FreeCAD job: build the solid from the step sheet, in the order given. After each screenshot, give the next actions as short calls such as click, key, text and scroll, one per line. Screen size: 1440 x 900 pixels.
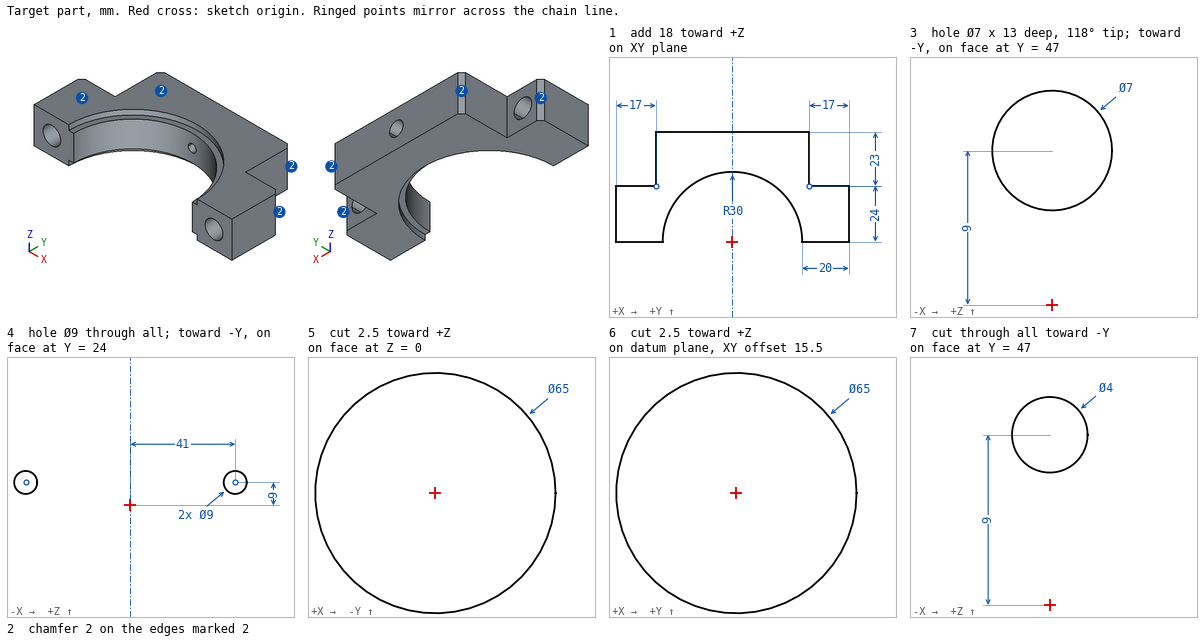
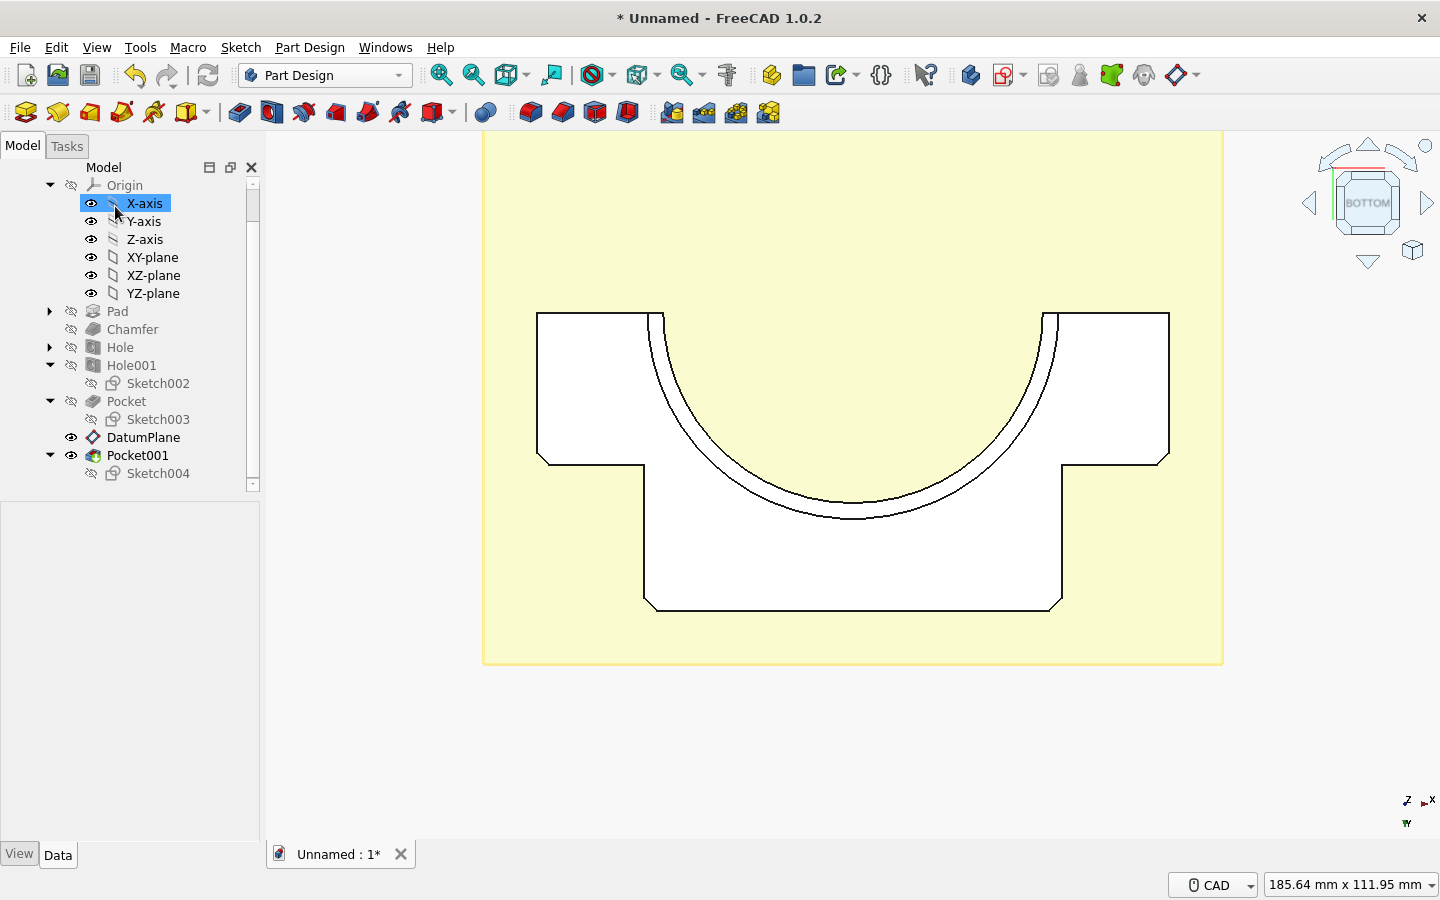
click(116, 437)
key(space)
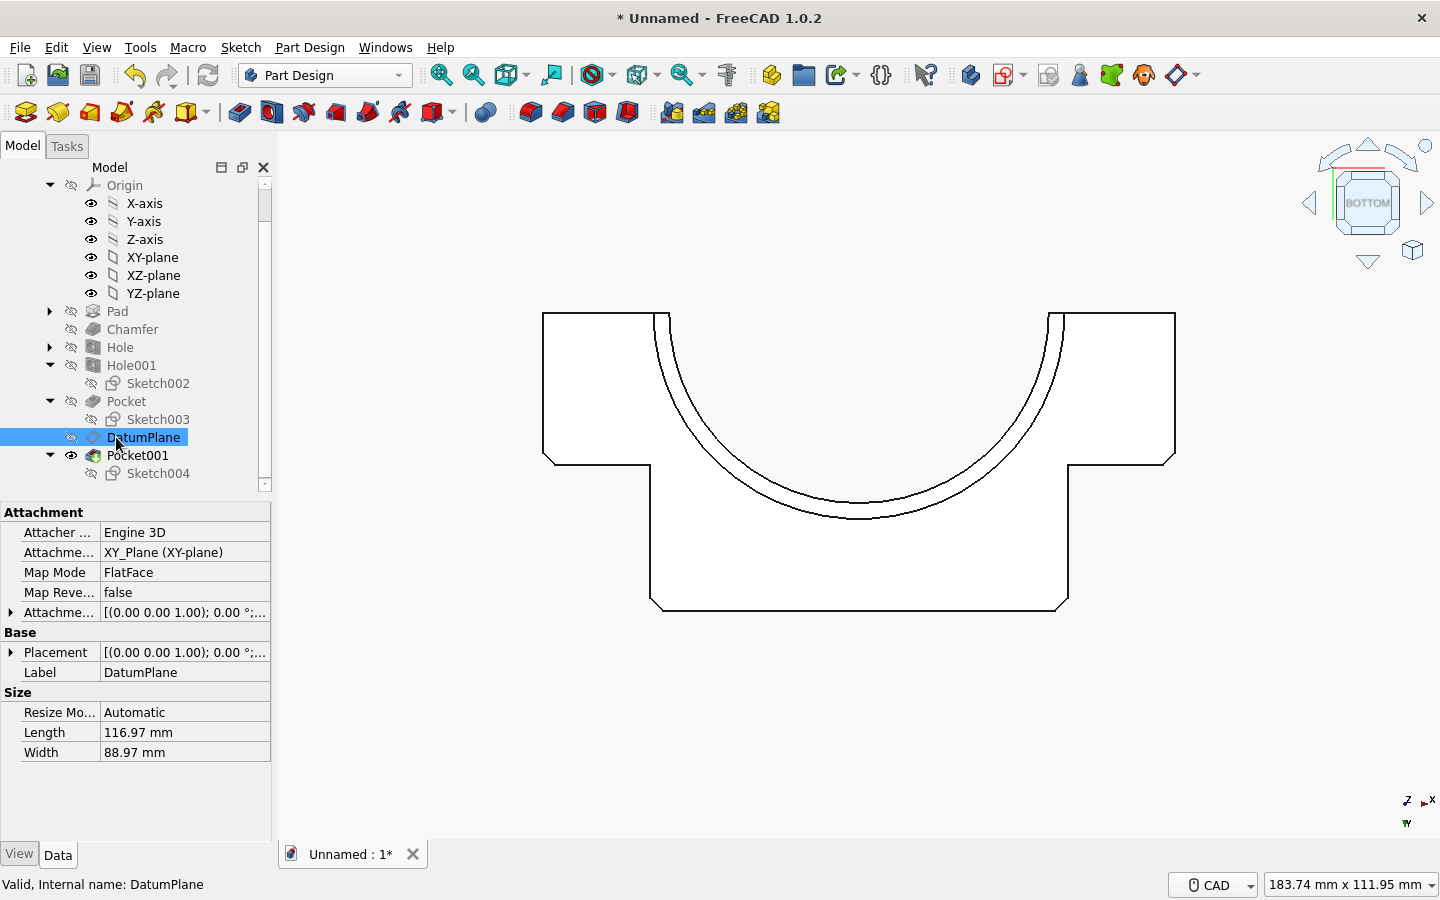
key(4)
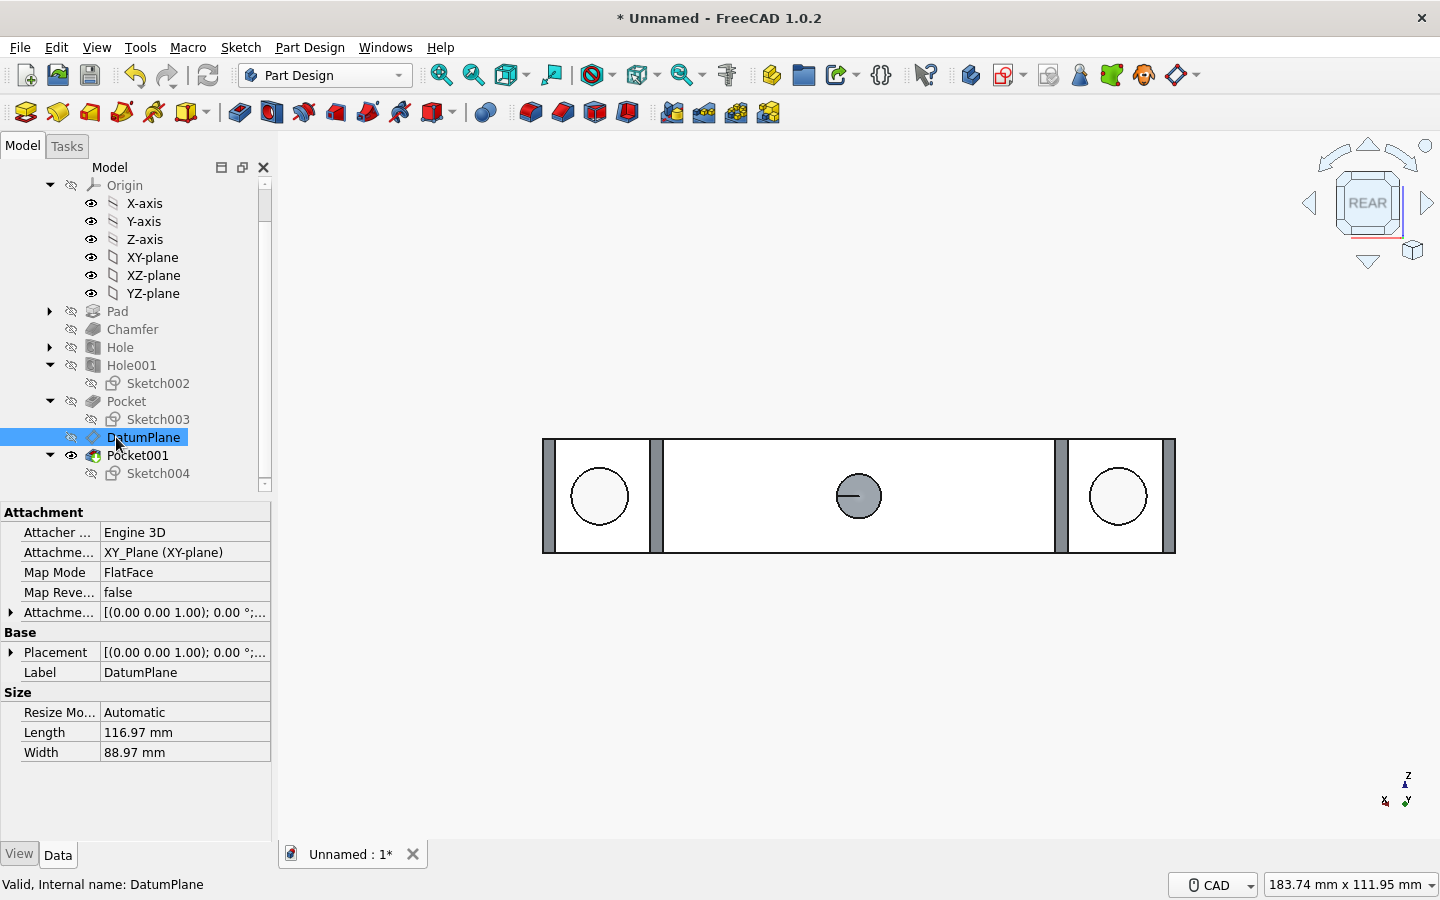
click(747, 495)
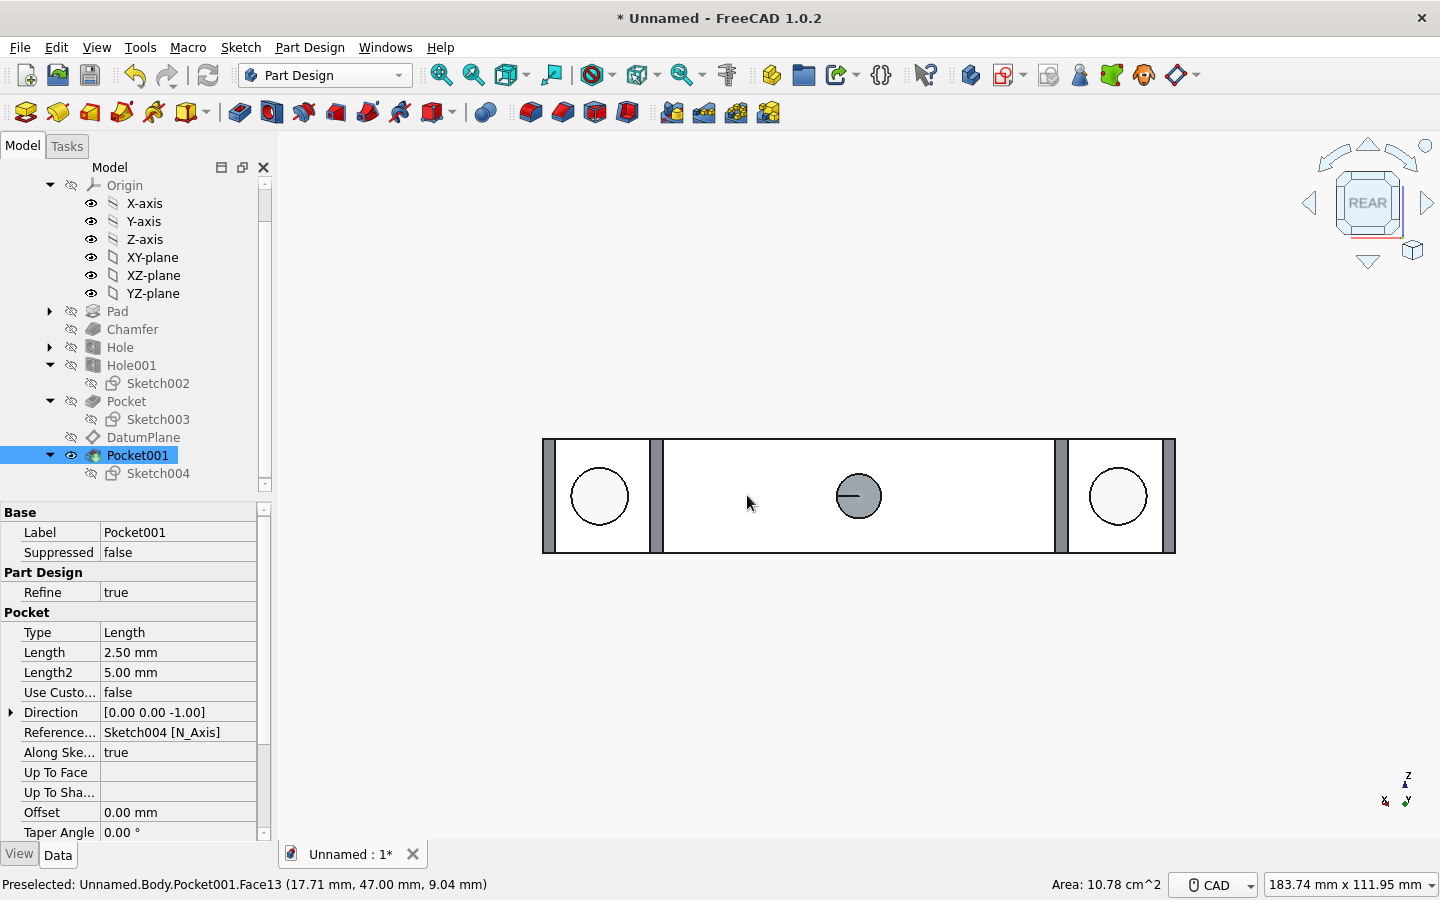
click(1004, 76)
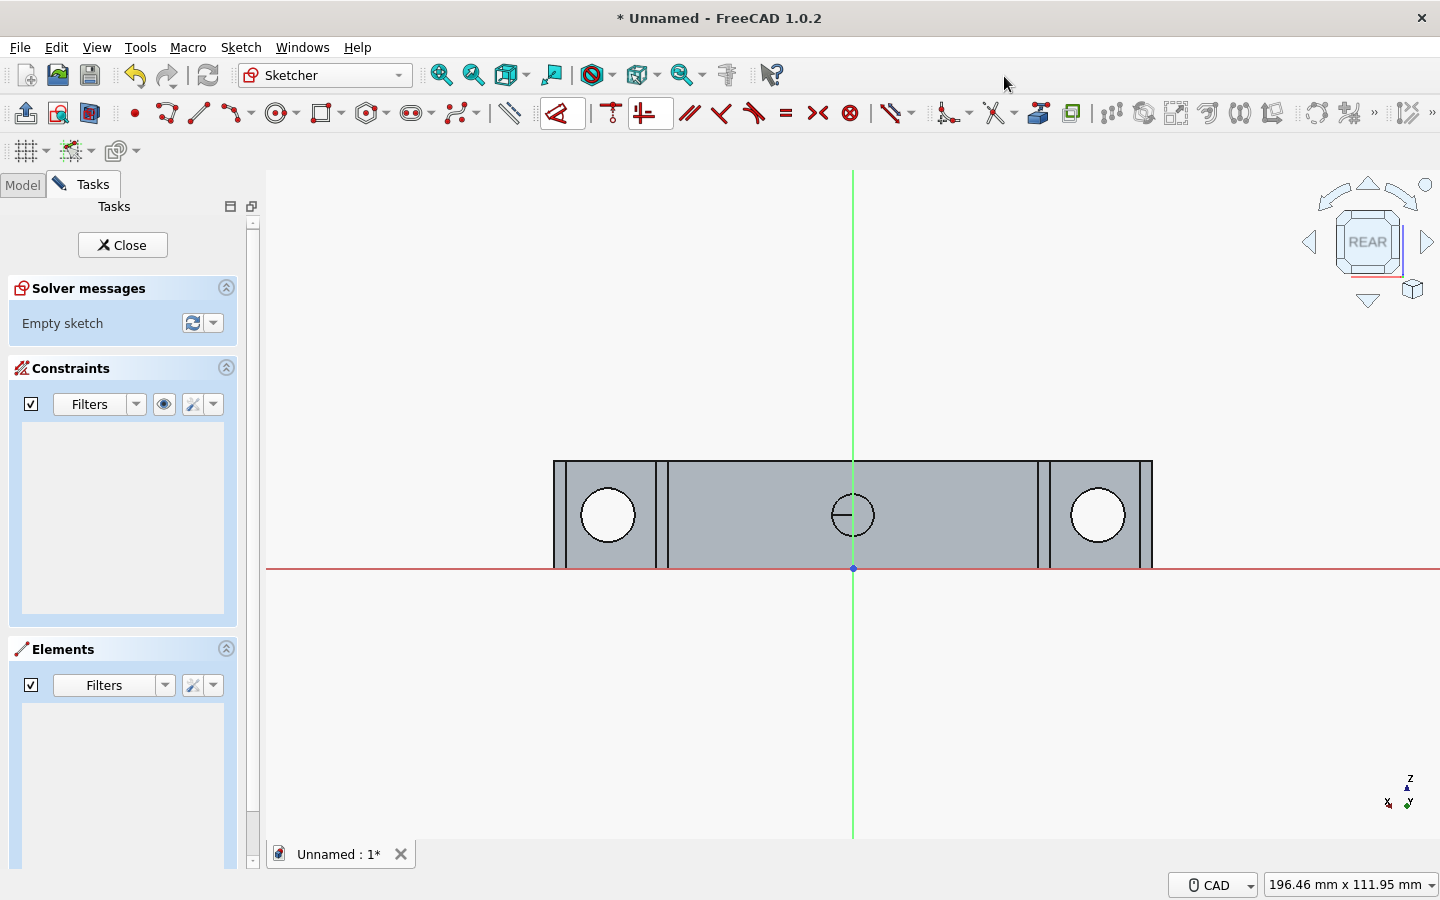
scroll(857, 516, up, 14)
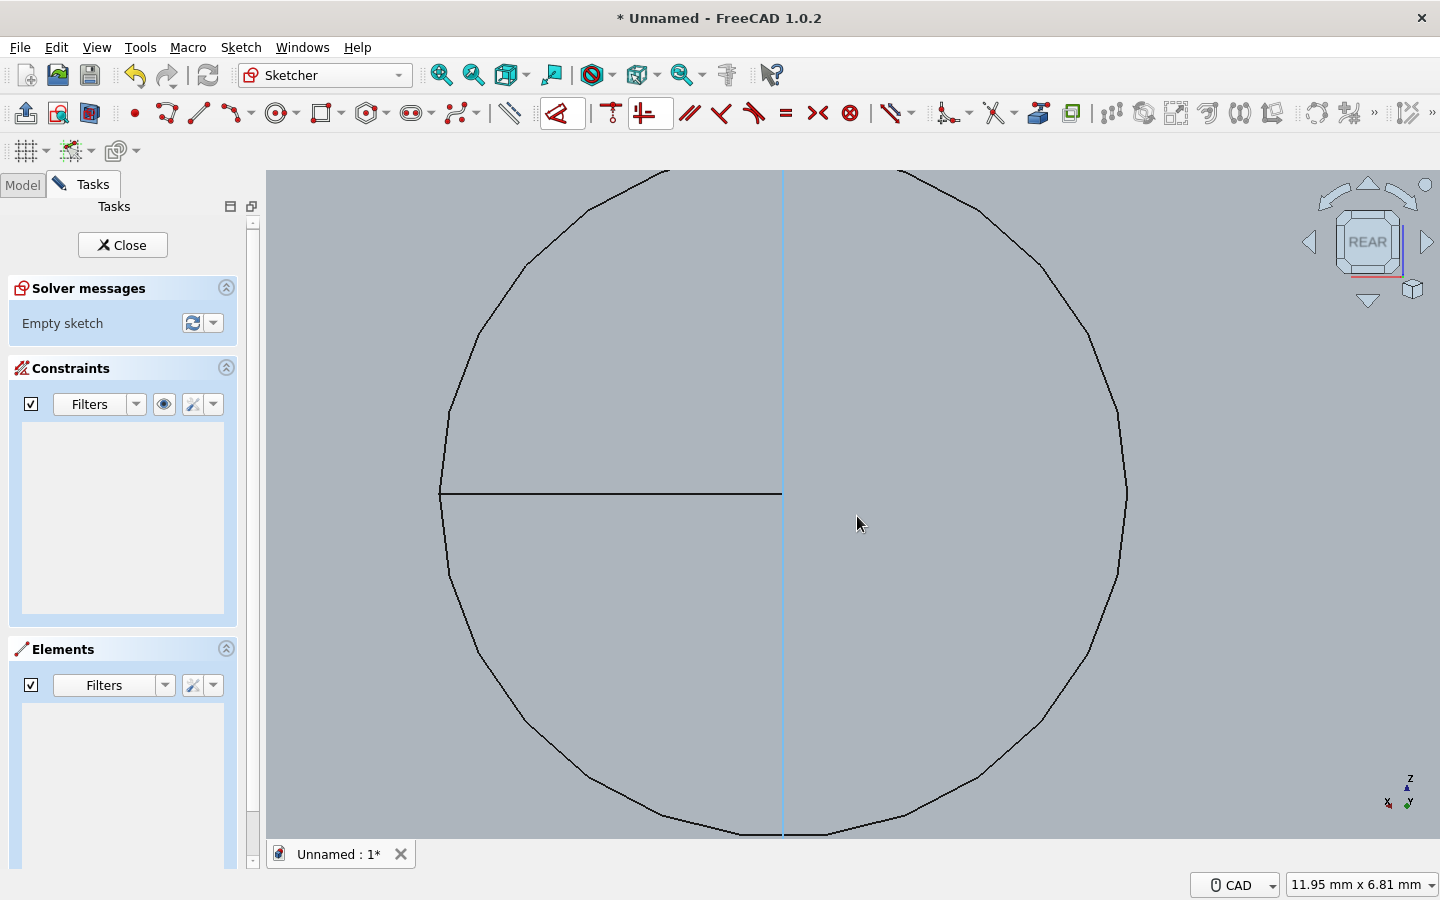
click(276, 114)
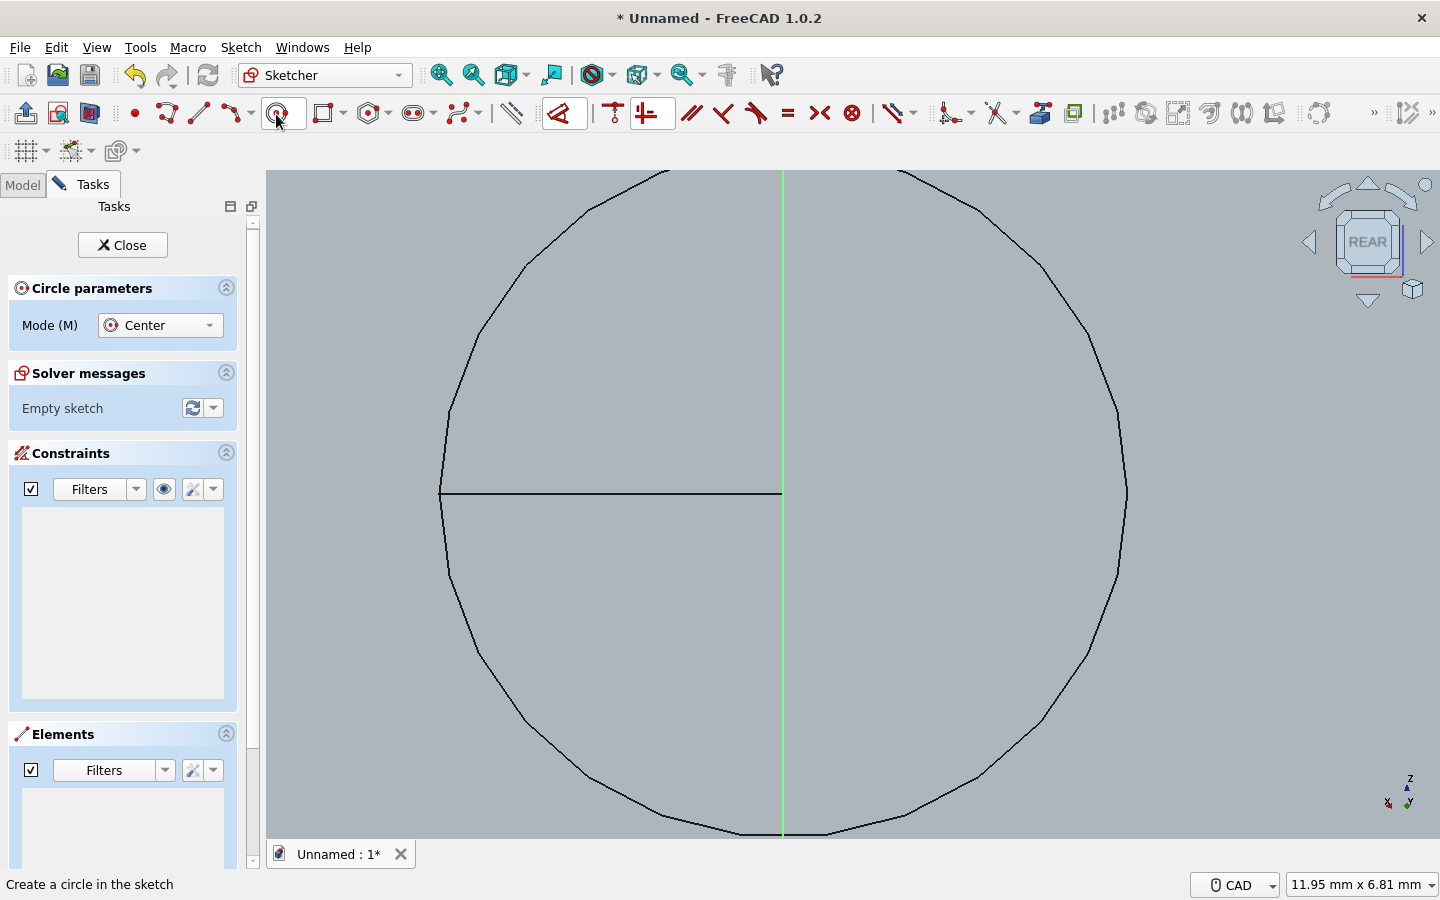
click(783, 494)
click(922, 355)
key(Escape)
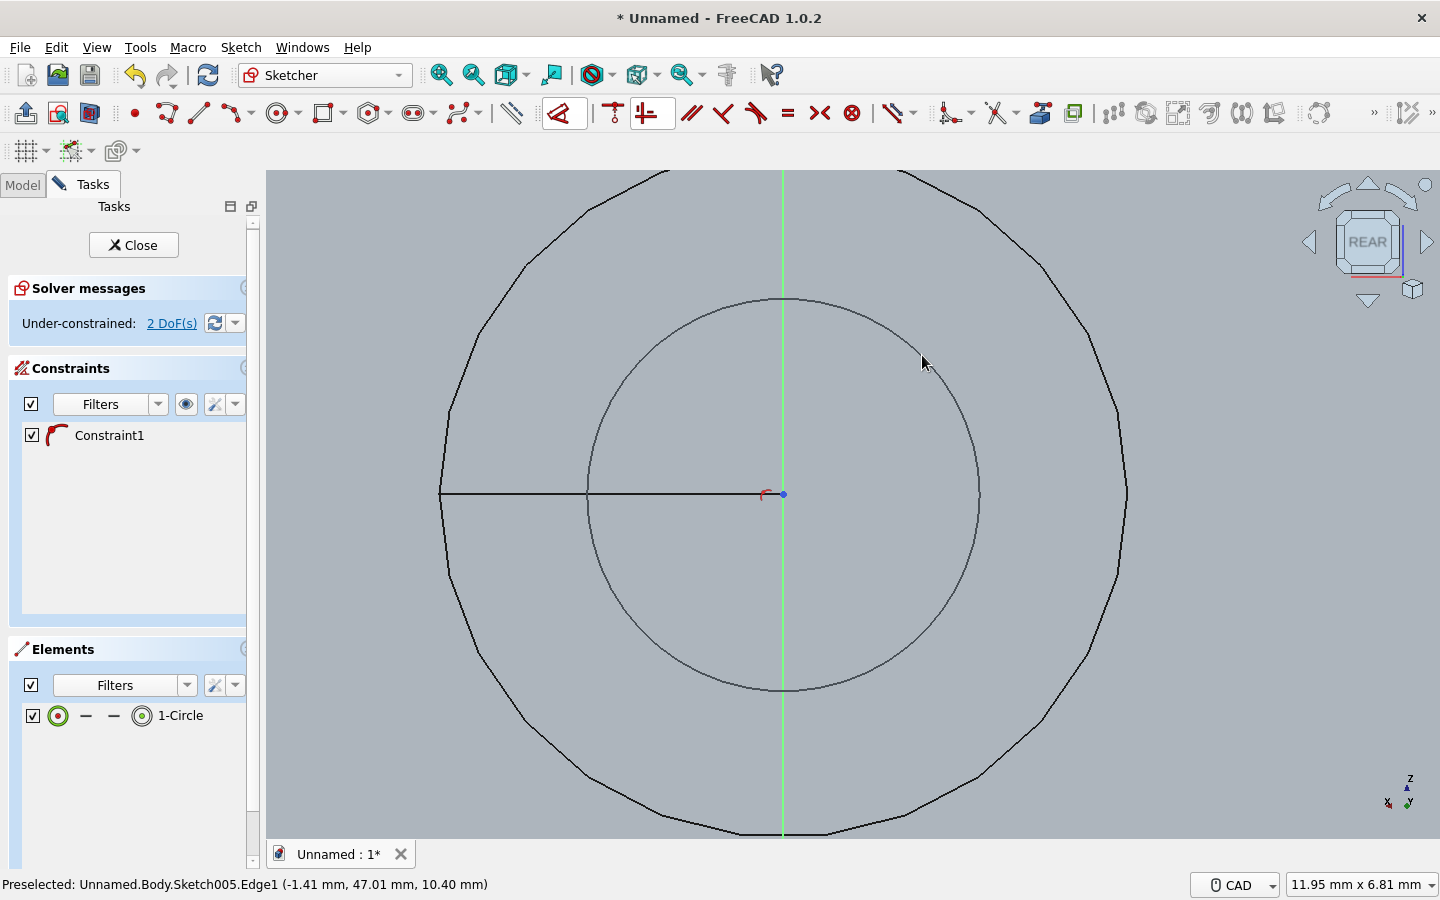
click(922, 356)